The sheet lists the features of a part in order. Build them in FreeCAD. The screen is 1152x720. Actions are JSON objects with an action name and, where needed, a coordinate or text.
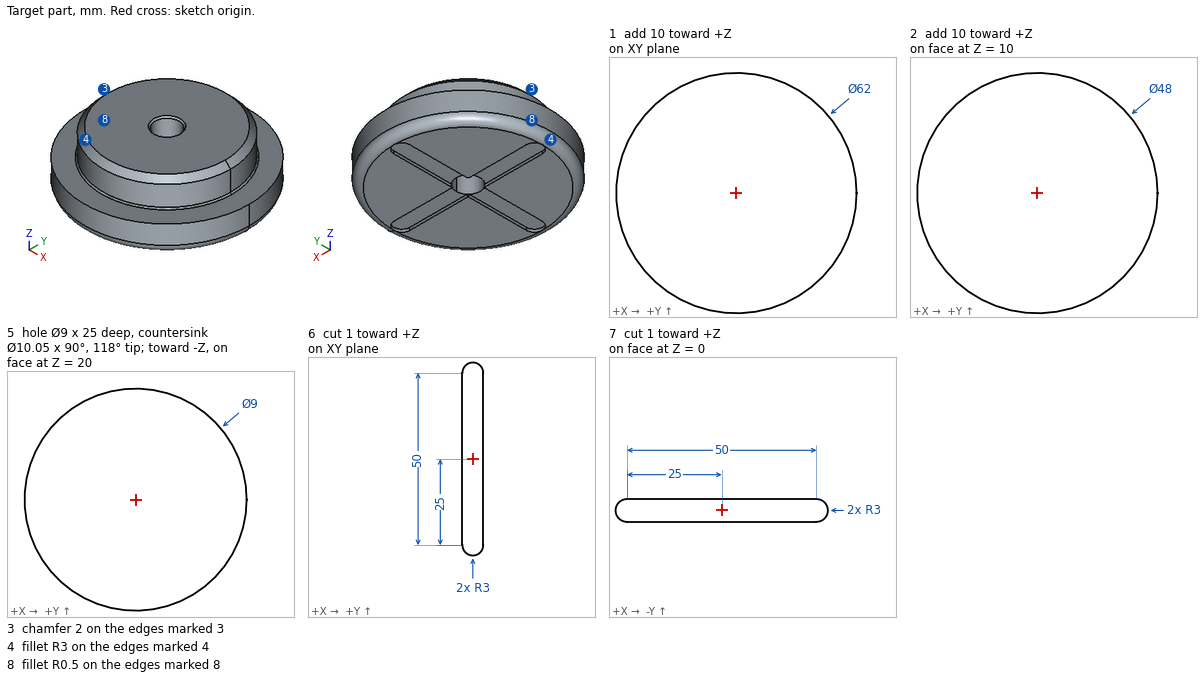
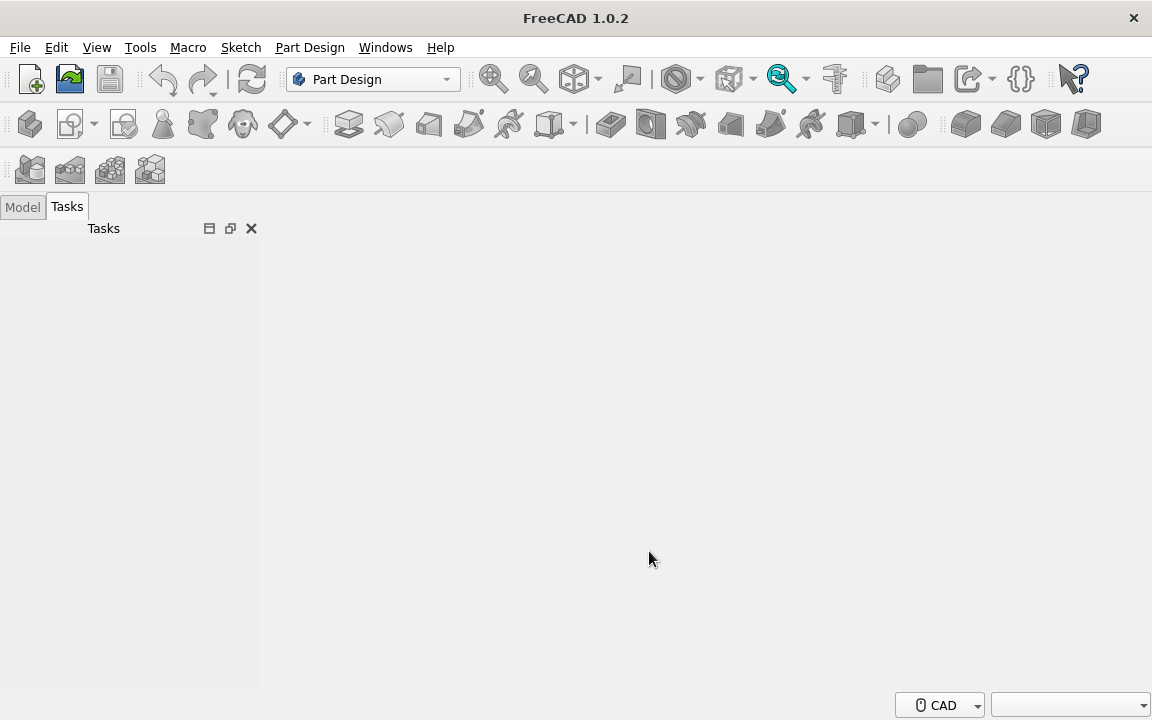
{"action": "left_click", "coordinate": [30, 80]}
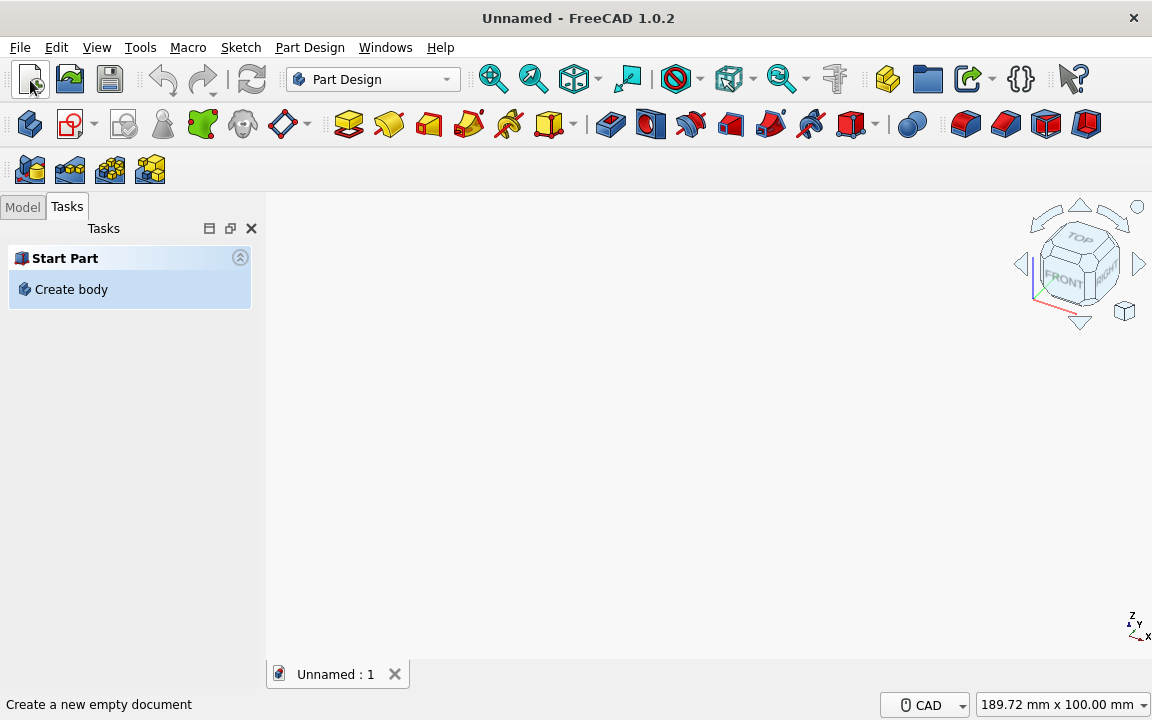
{"action": "left_click", "coordinate": [70, 124]}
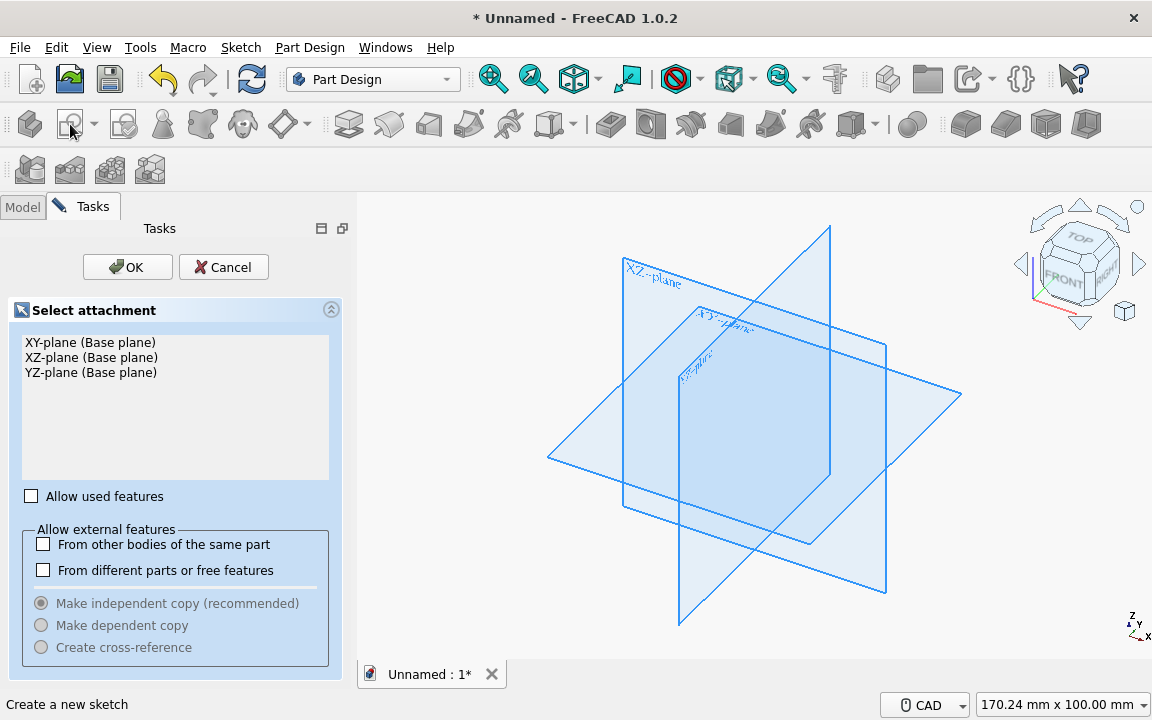
{"action": "left_click", "coordinate": [82, 342]}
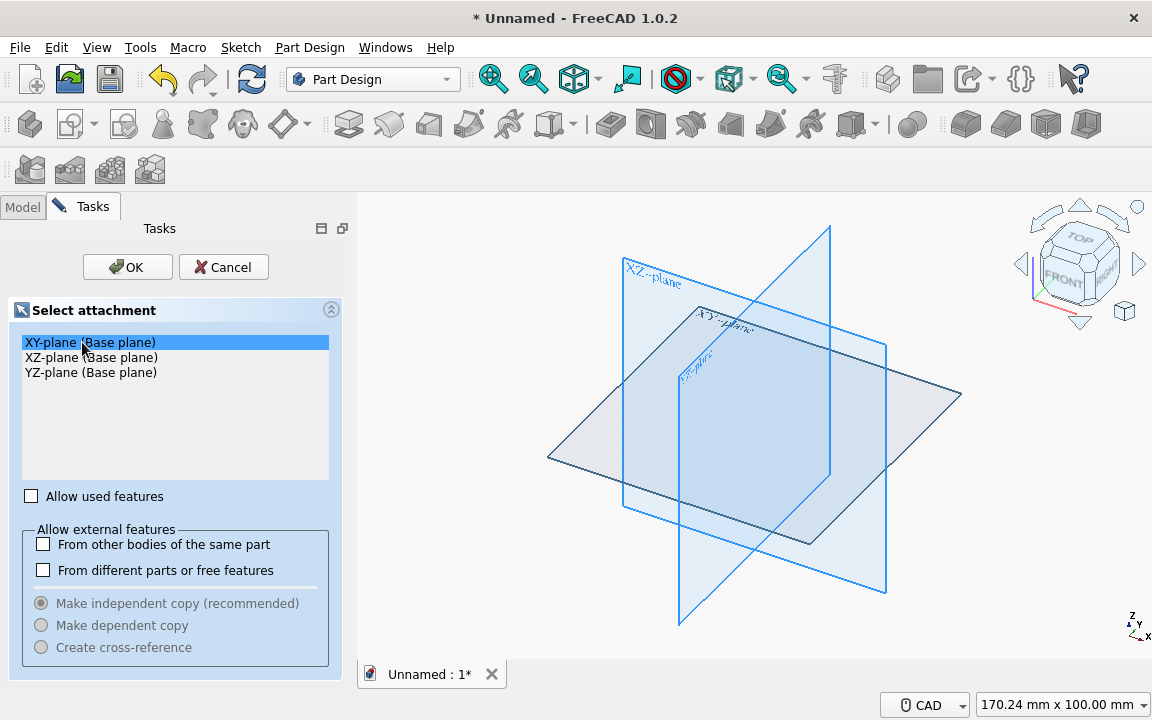
{"action": "left_click", "coordinate": [128, 267]}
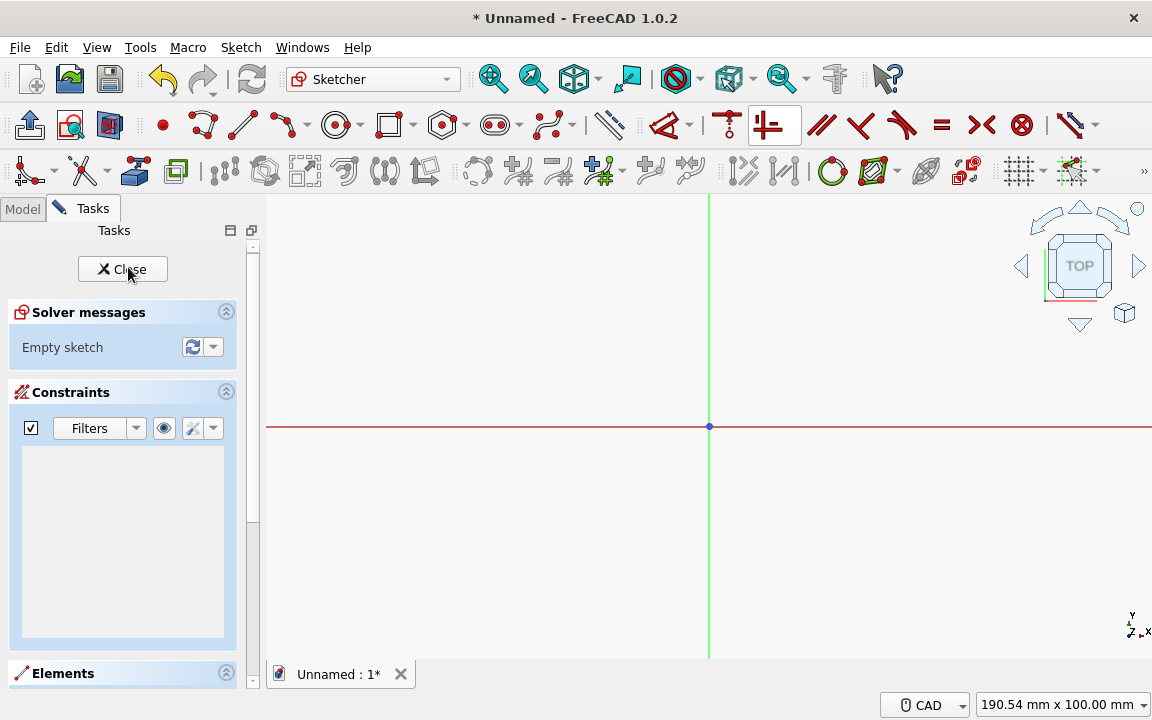
{"action": "key", "text": "g c"}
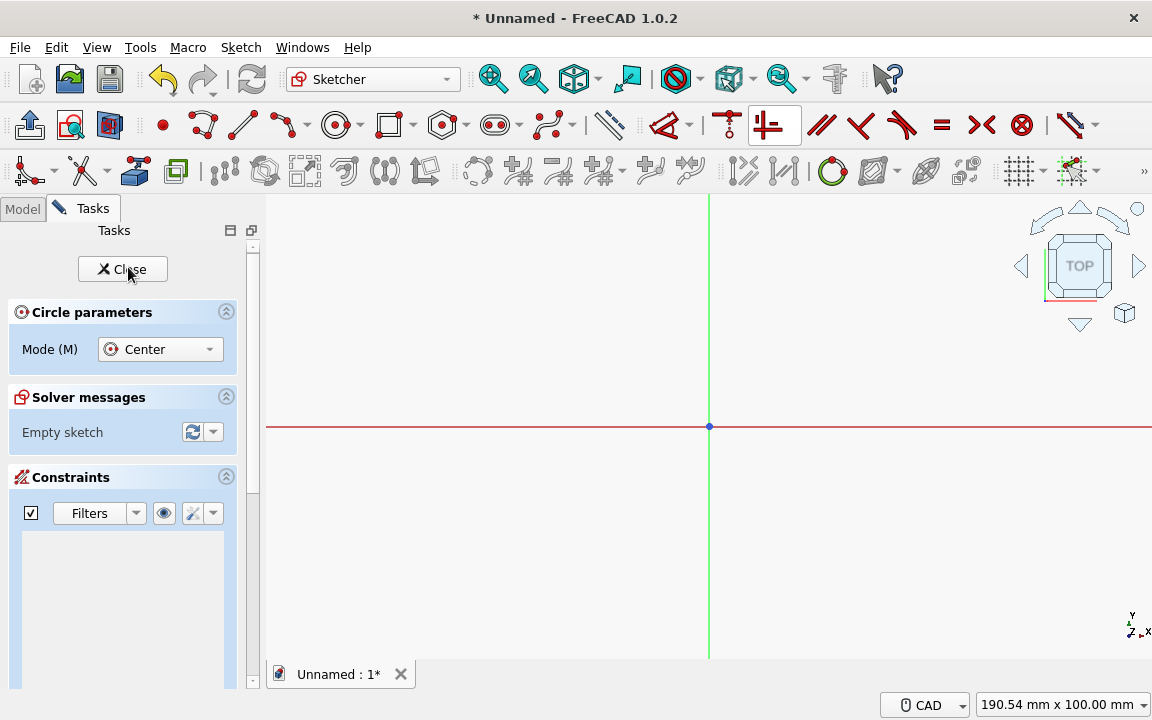
{"action": "left_click", "coordinate": [709, 426]}
{"action": "left_click", "coordinate": [811, 325]}
{"action": "key", "text": "Escape"}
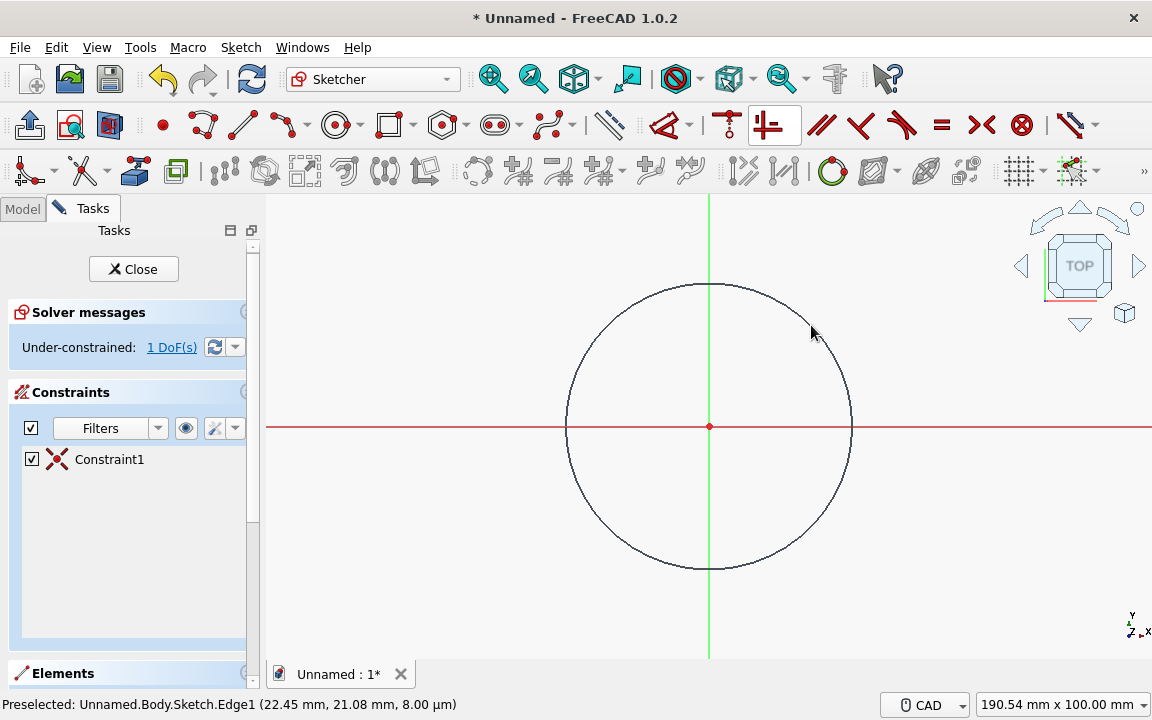
{"action": "left_click", "coordinate": [664, 126]}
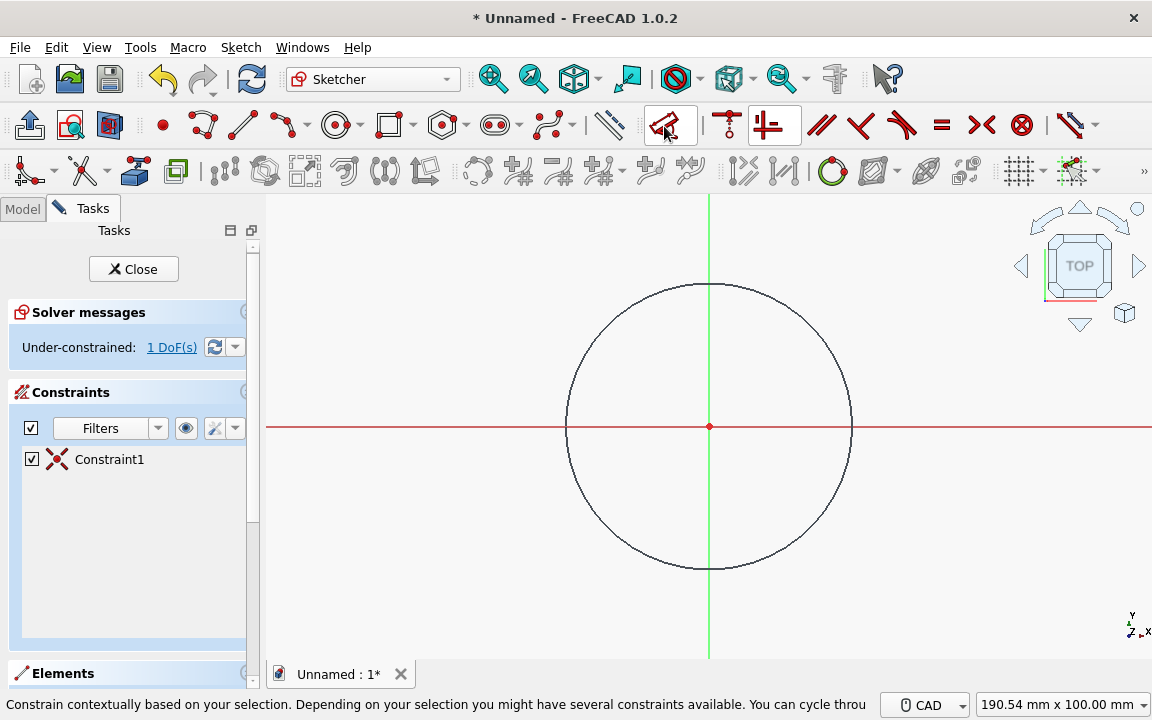
{"action": "left_click", "coordinate": [810, 325]}
{"action": "left_click", "coordinate": [833, 302]}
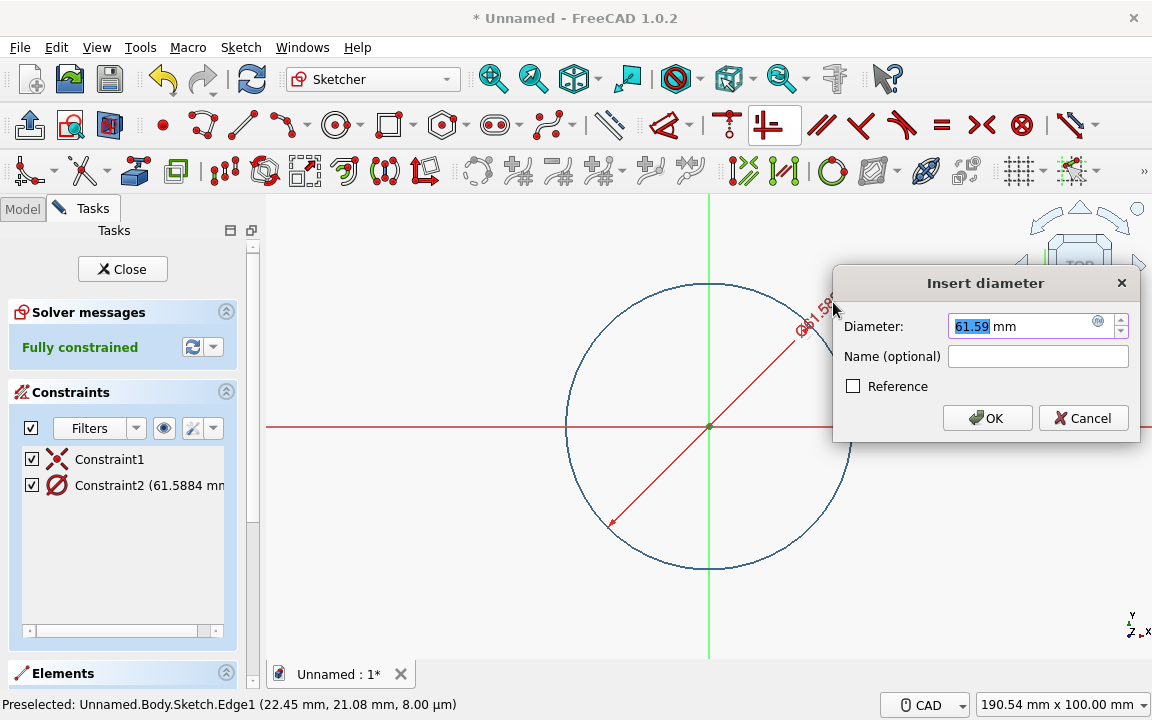
{"action": "type", "text": "62"}
{"action": "key", "text": "Return"}
{"action": "key", "text": "Escape"}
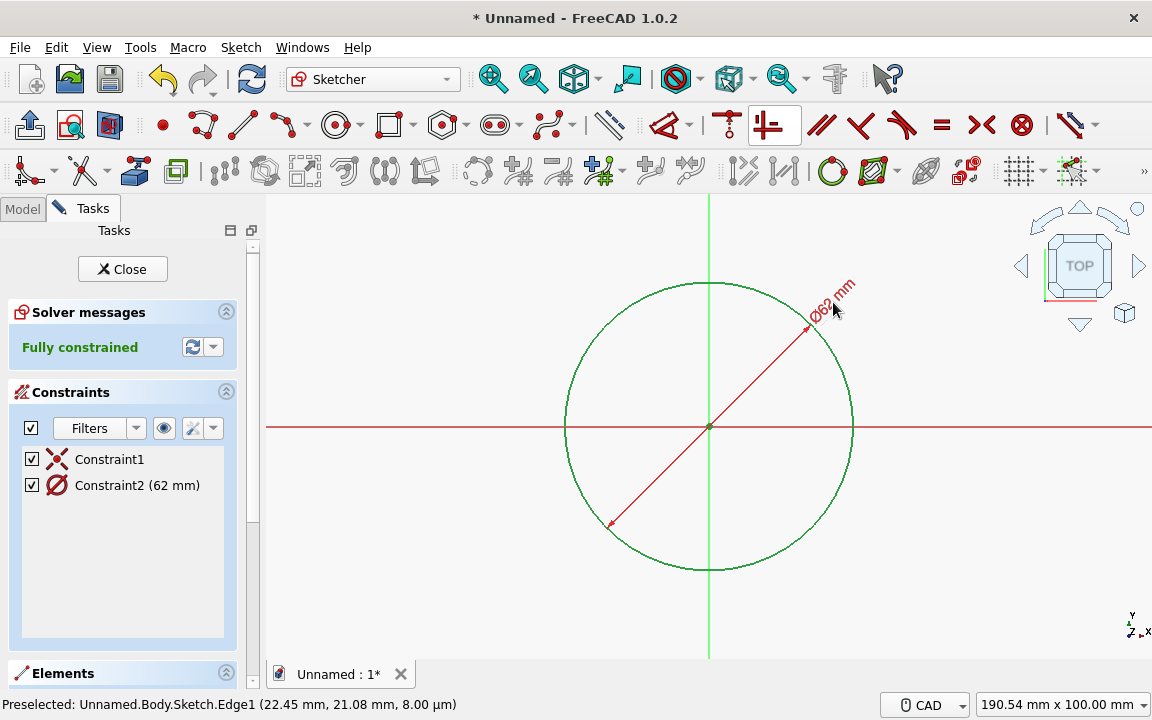
{"action": "left_click", "coordinate": [123, 269]}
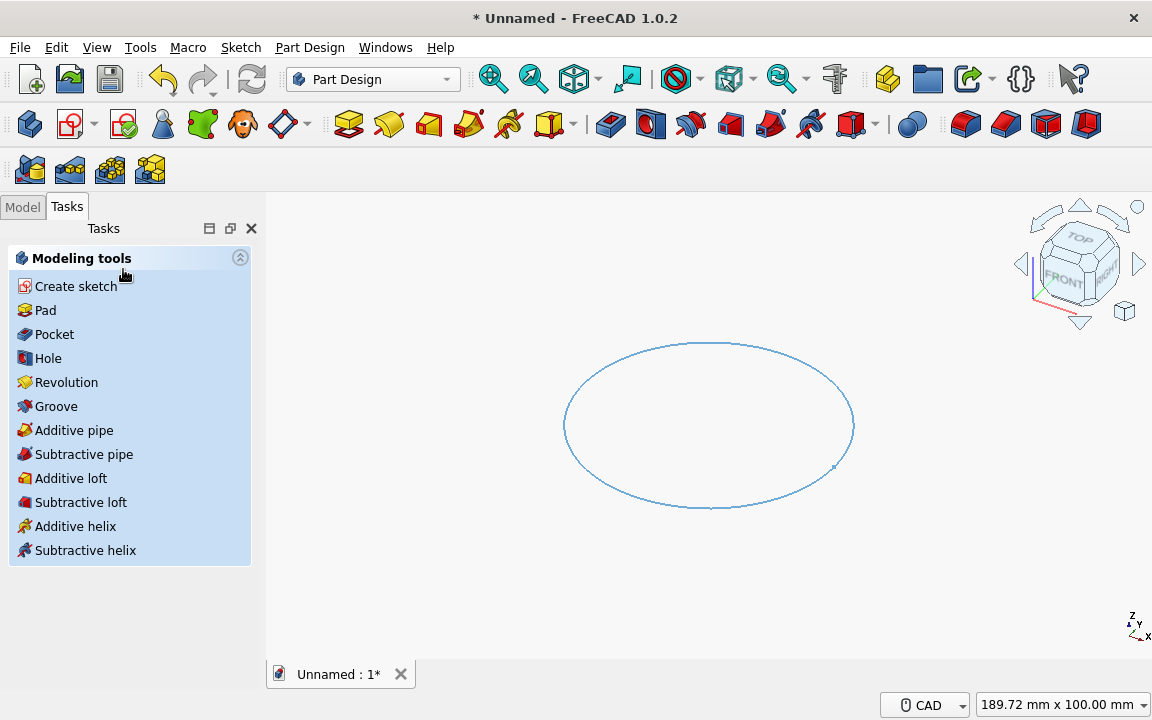
{"action": "left_click", "coordinate": [350, 124]}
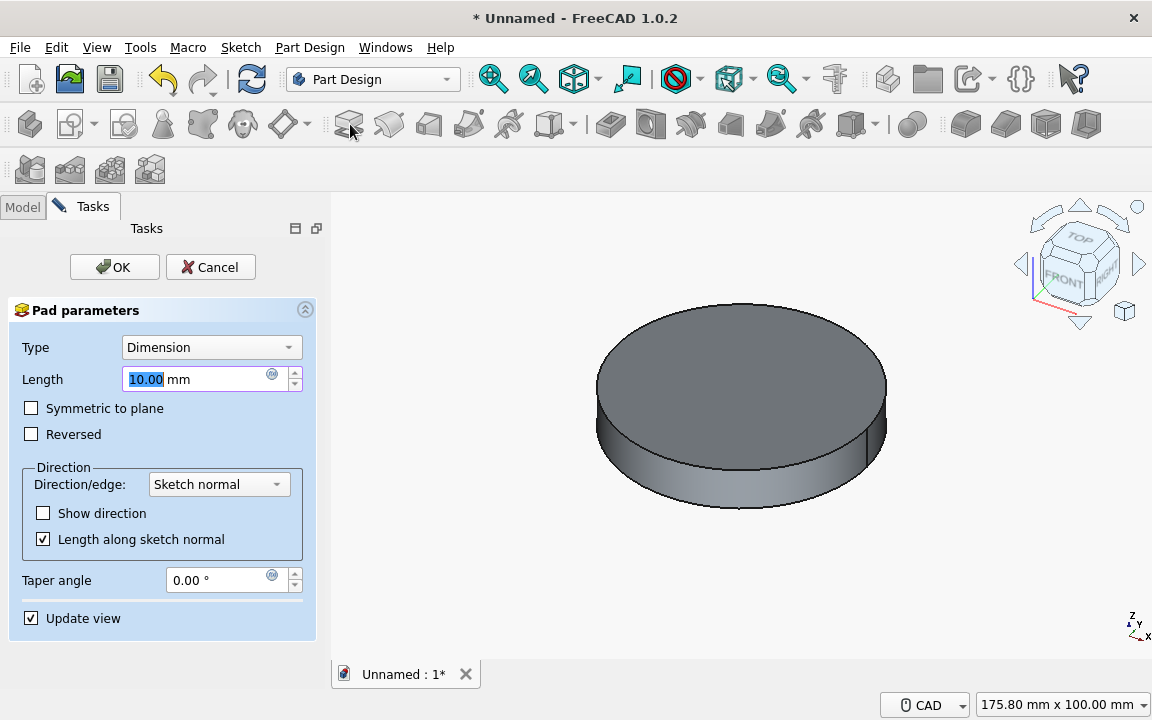
{"action": "type", "text": "10"}
{"action": "key", "text": "Tab"}